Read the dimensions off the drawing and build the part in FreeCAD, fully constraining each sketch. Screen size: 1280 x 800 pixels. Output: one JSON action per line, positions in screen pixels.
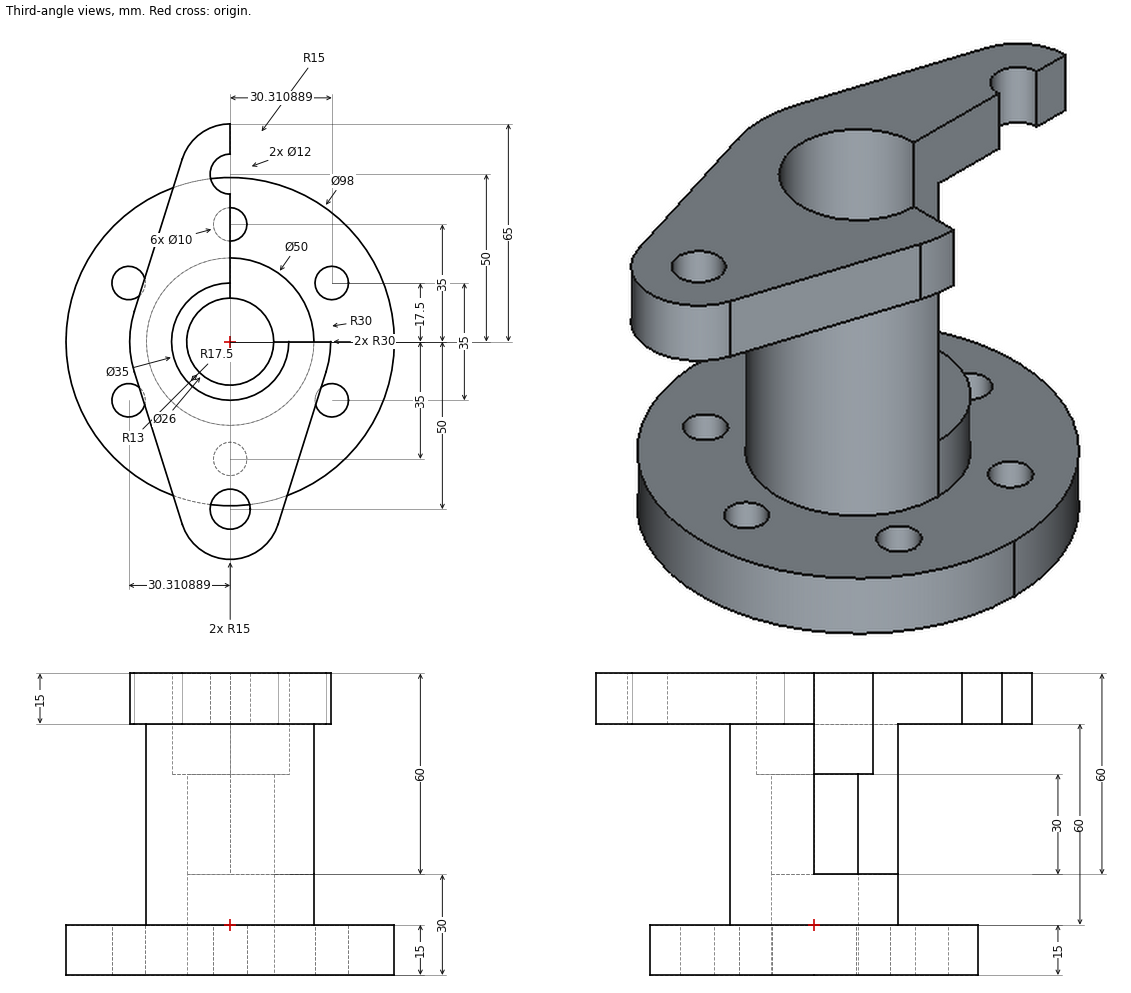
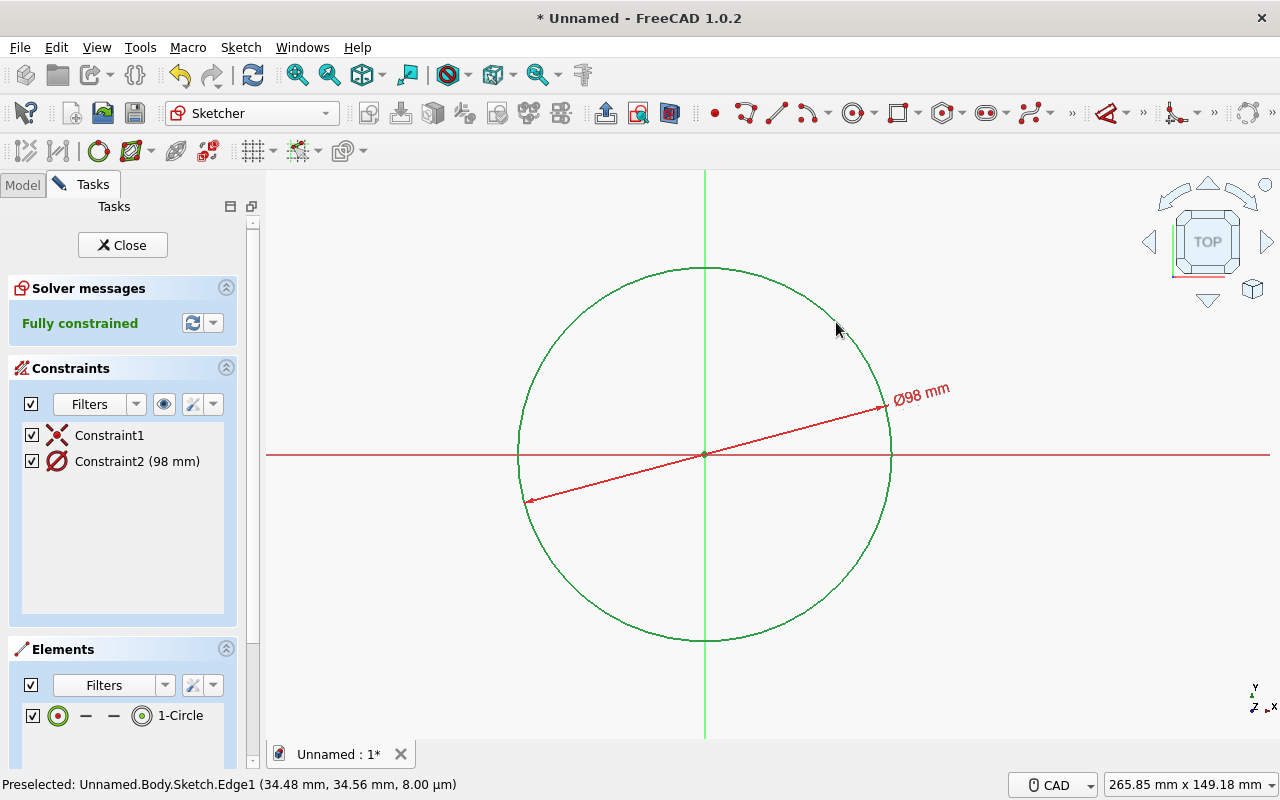
{"action": "left_click", "coordinate": [123, 245]}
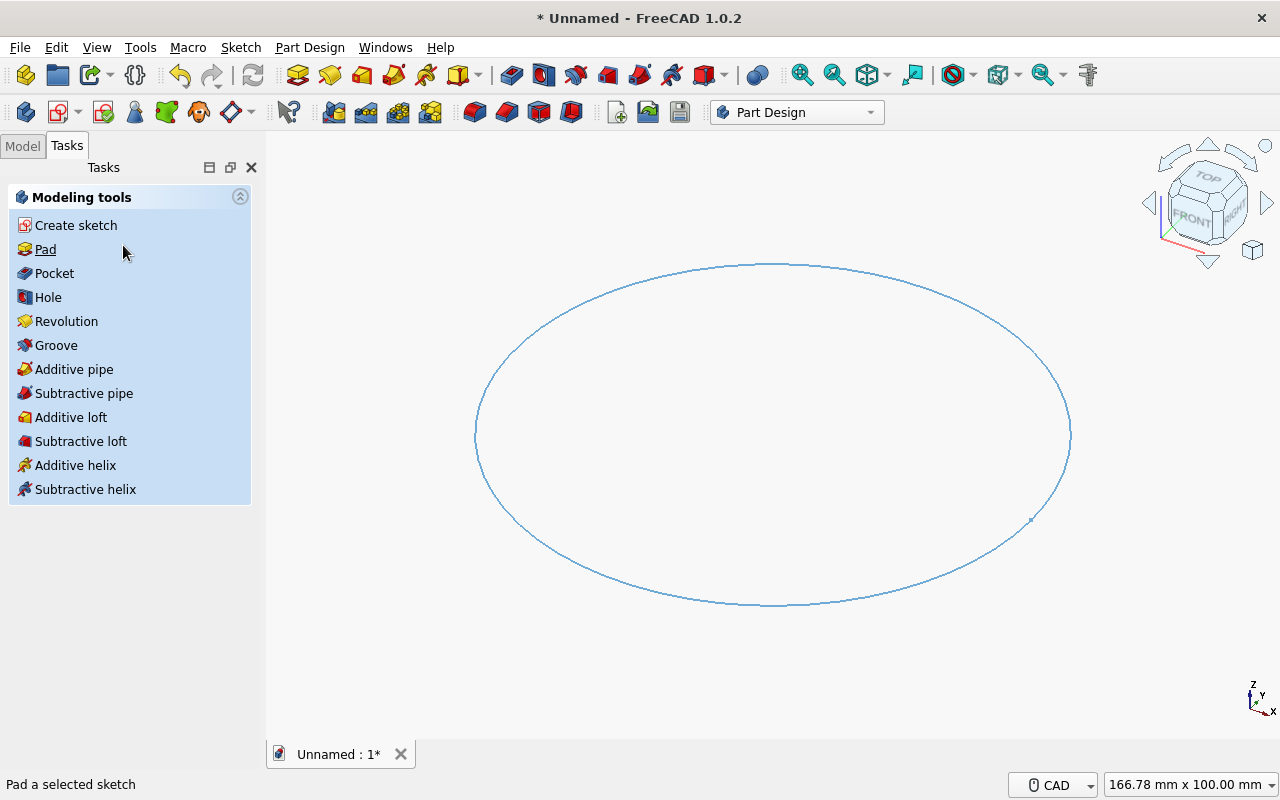
{"action": "left_click", "coordinate": [298, 76]}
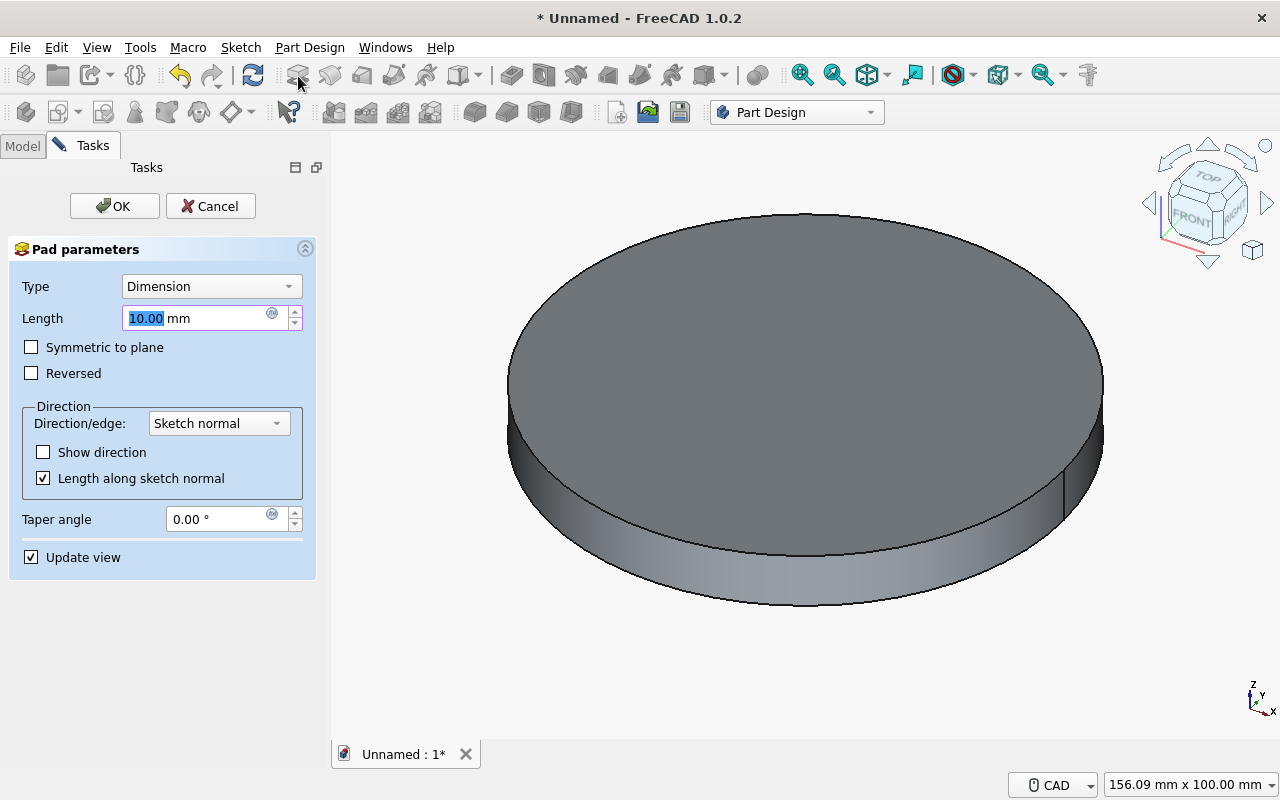
{"action": "type", "text": "15"}
{"action": "key", "text": "Tab"}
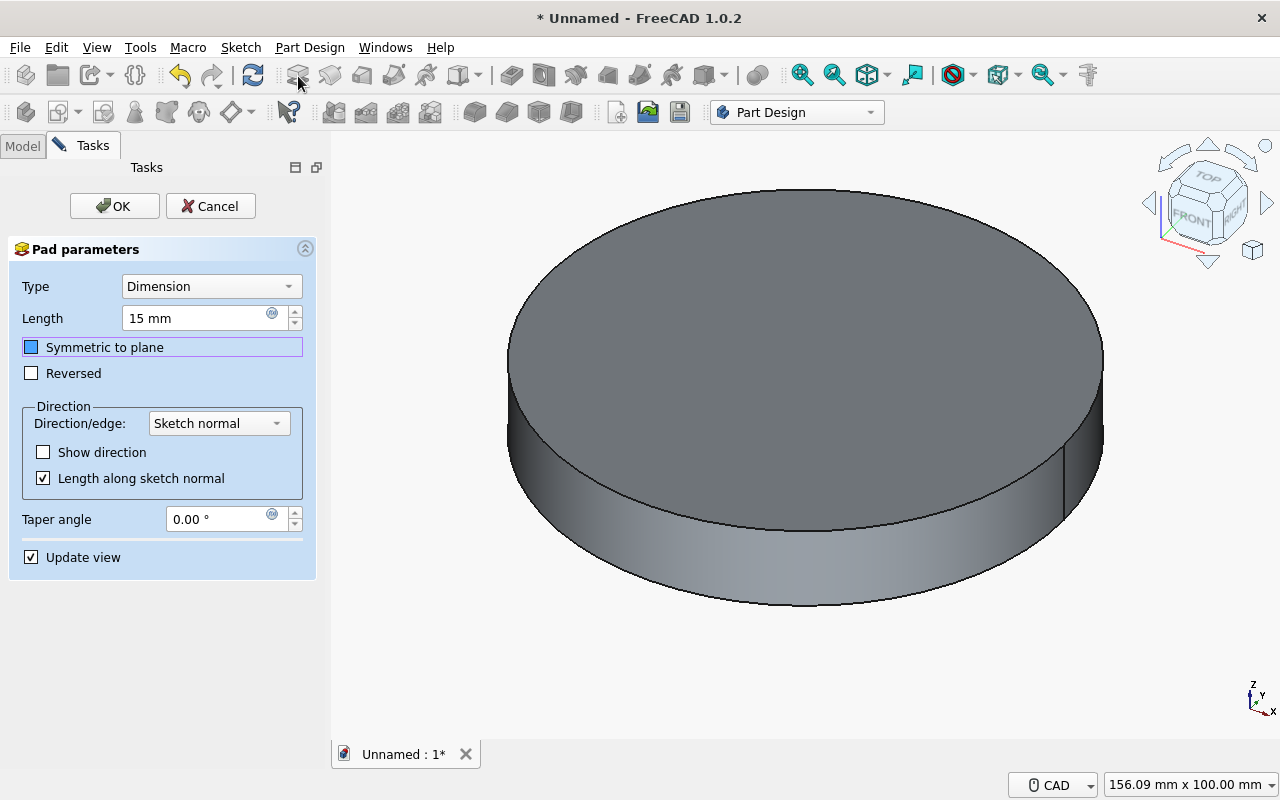
{"action": "left_click", "coordinate": [30, 373]}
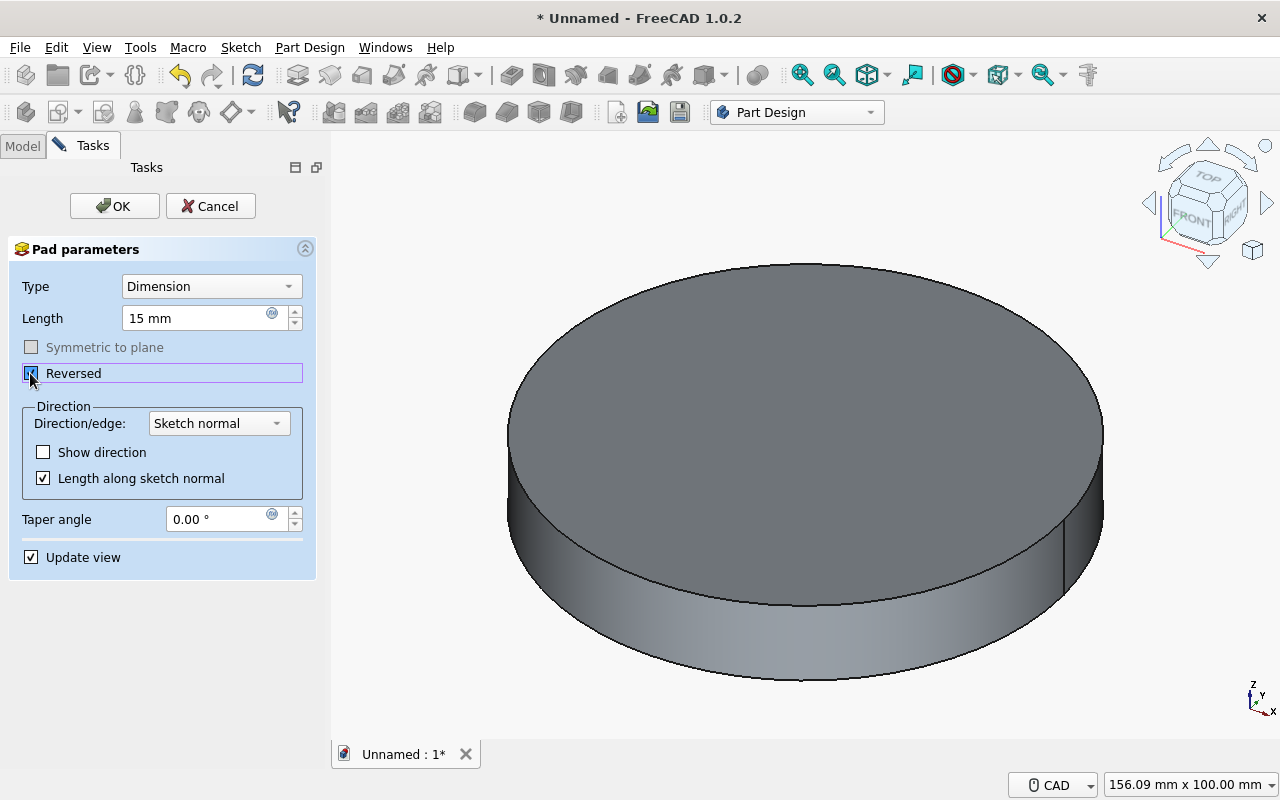
{"action": "left_click", "coordinate": [115, 206]}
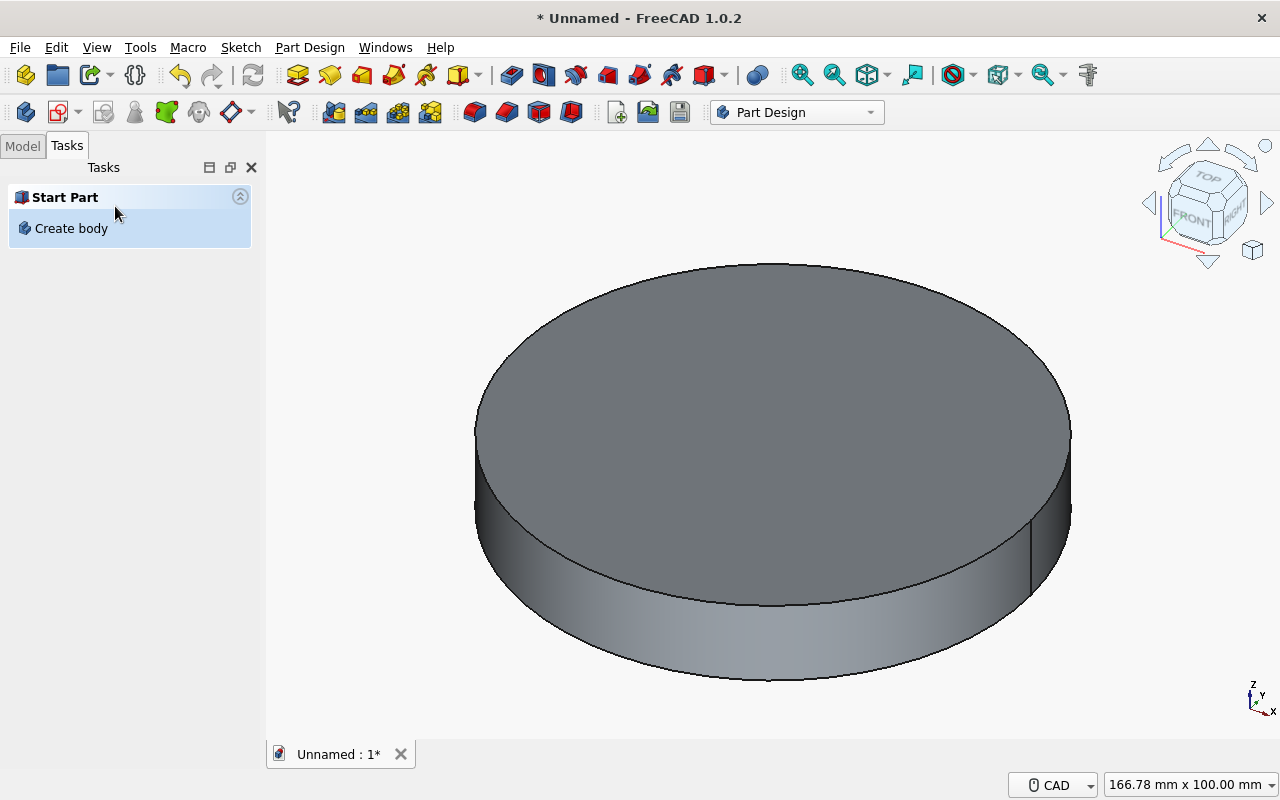
{"action": "key", "text": "v f"}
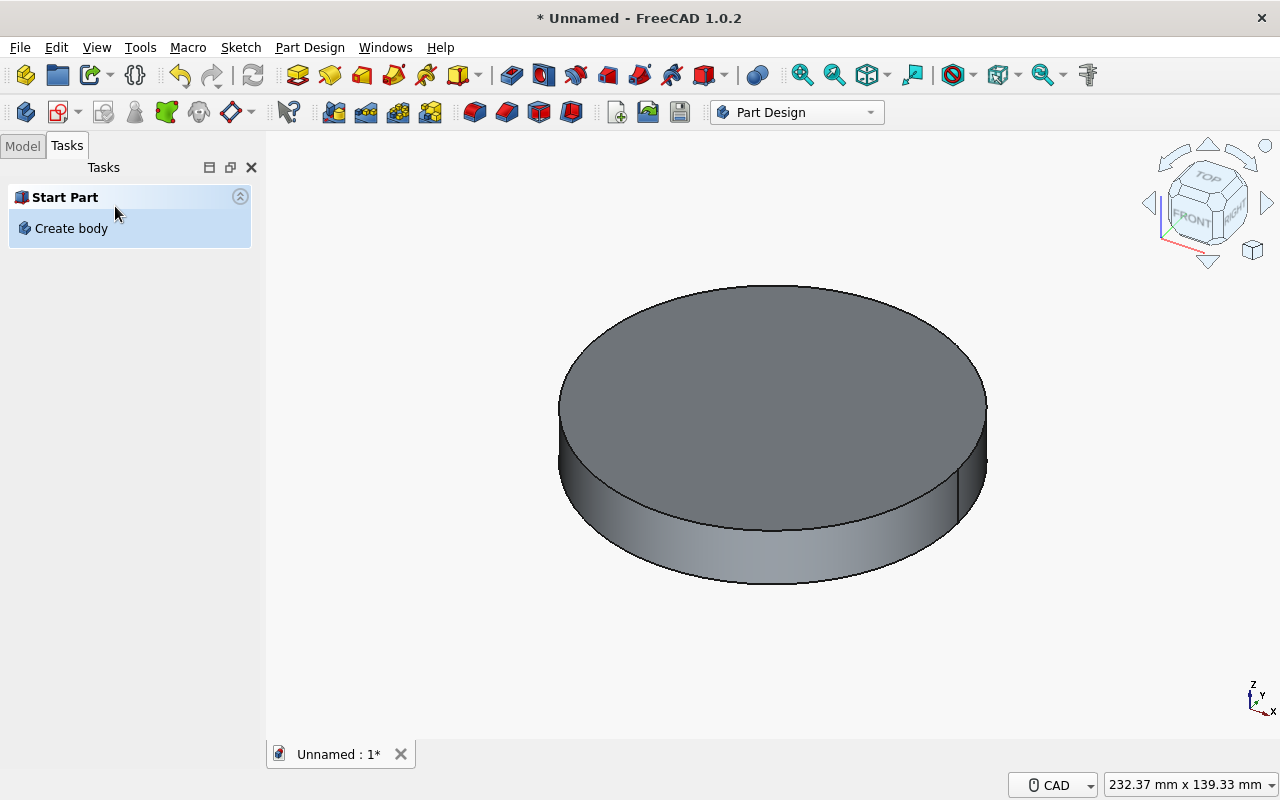
{"action": "left_click", "coordinate": [773, 407]}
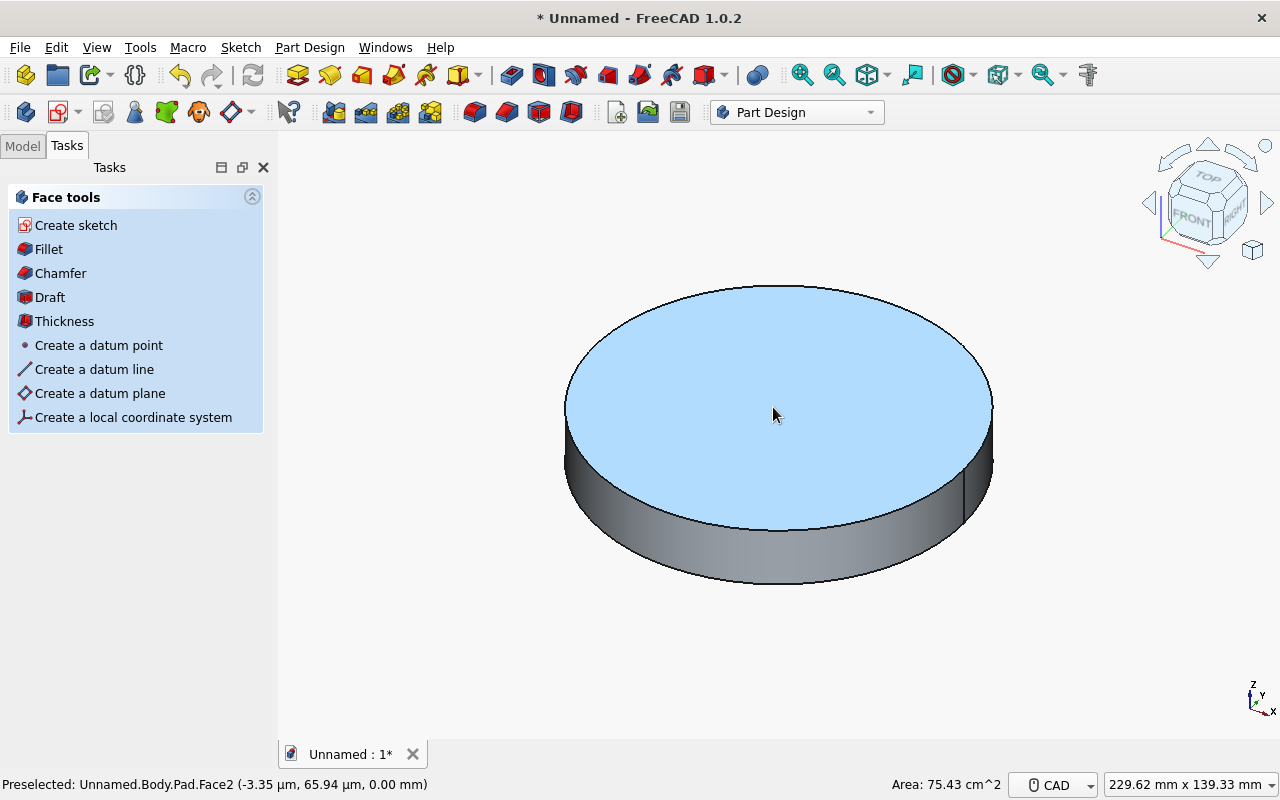
{"action": "left_click", "coordinate": [58, 112]}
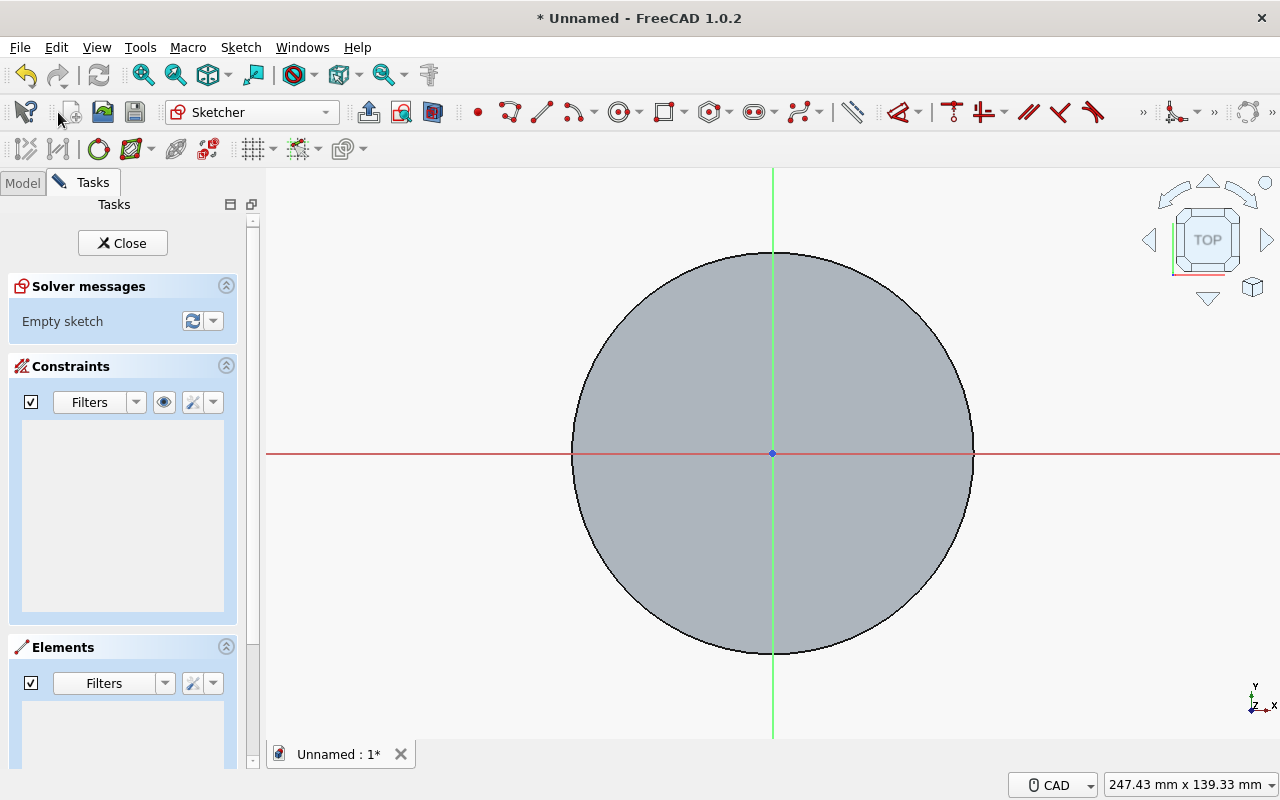
{"action": "key", "text": "g c"}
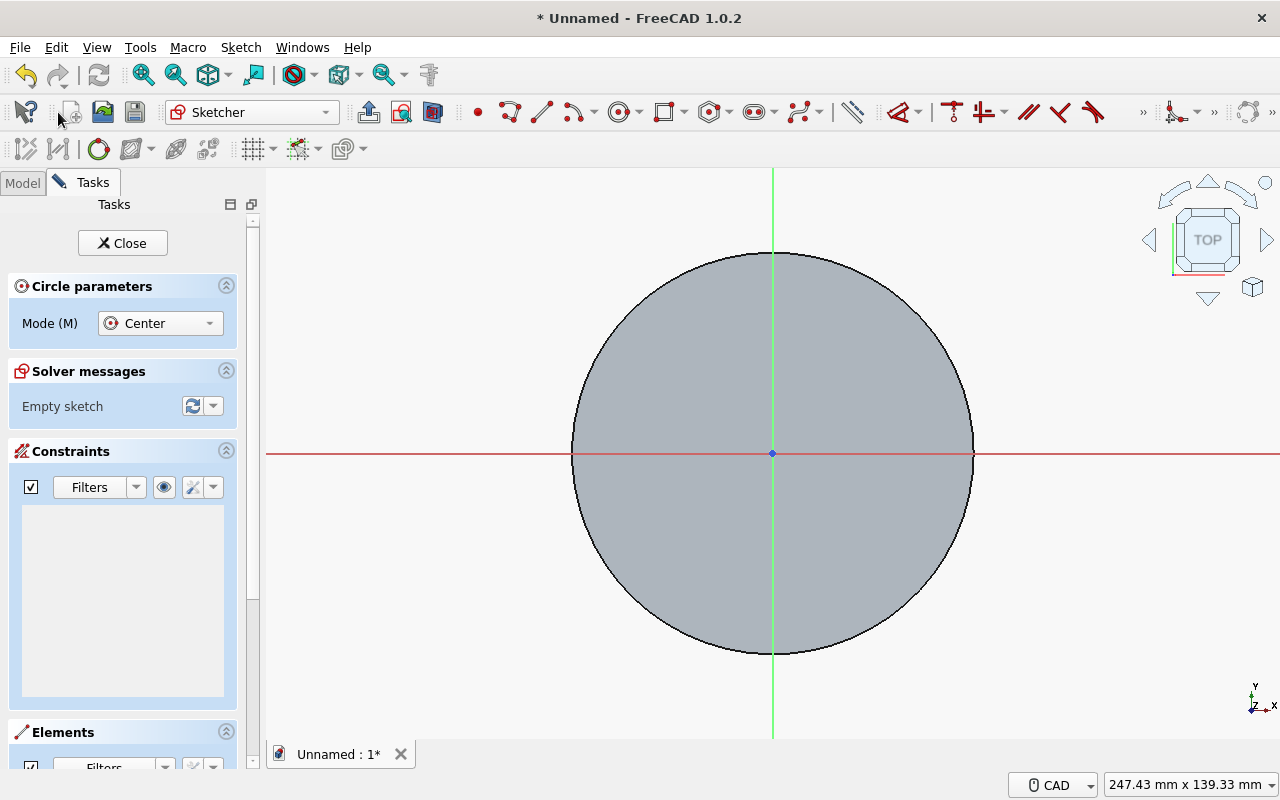
{"action": "left_click", "coordinate": [773, 310]}
{"action": "left_click", "coordinate": [787, 296]}